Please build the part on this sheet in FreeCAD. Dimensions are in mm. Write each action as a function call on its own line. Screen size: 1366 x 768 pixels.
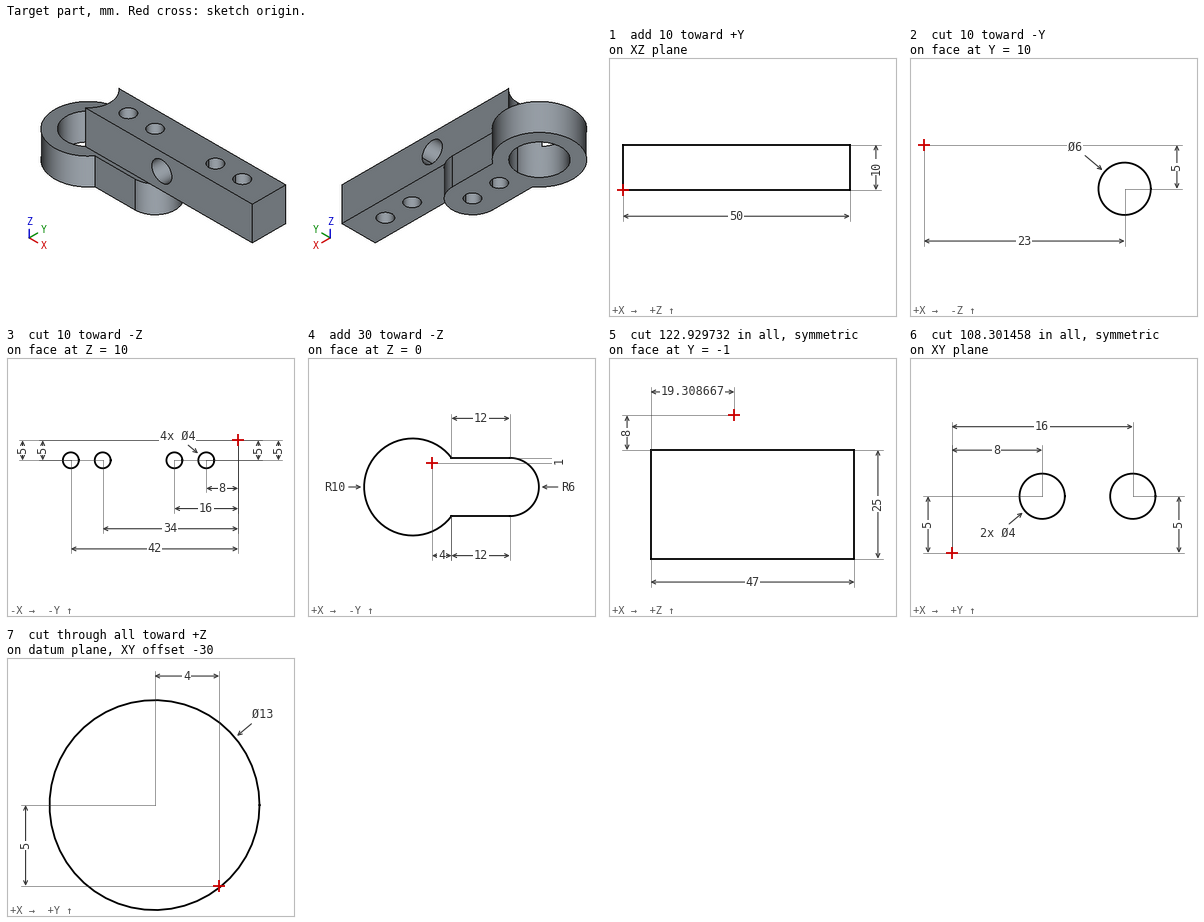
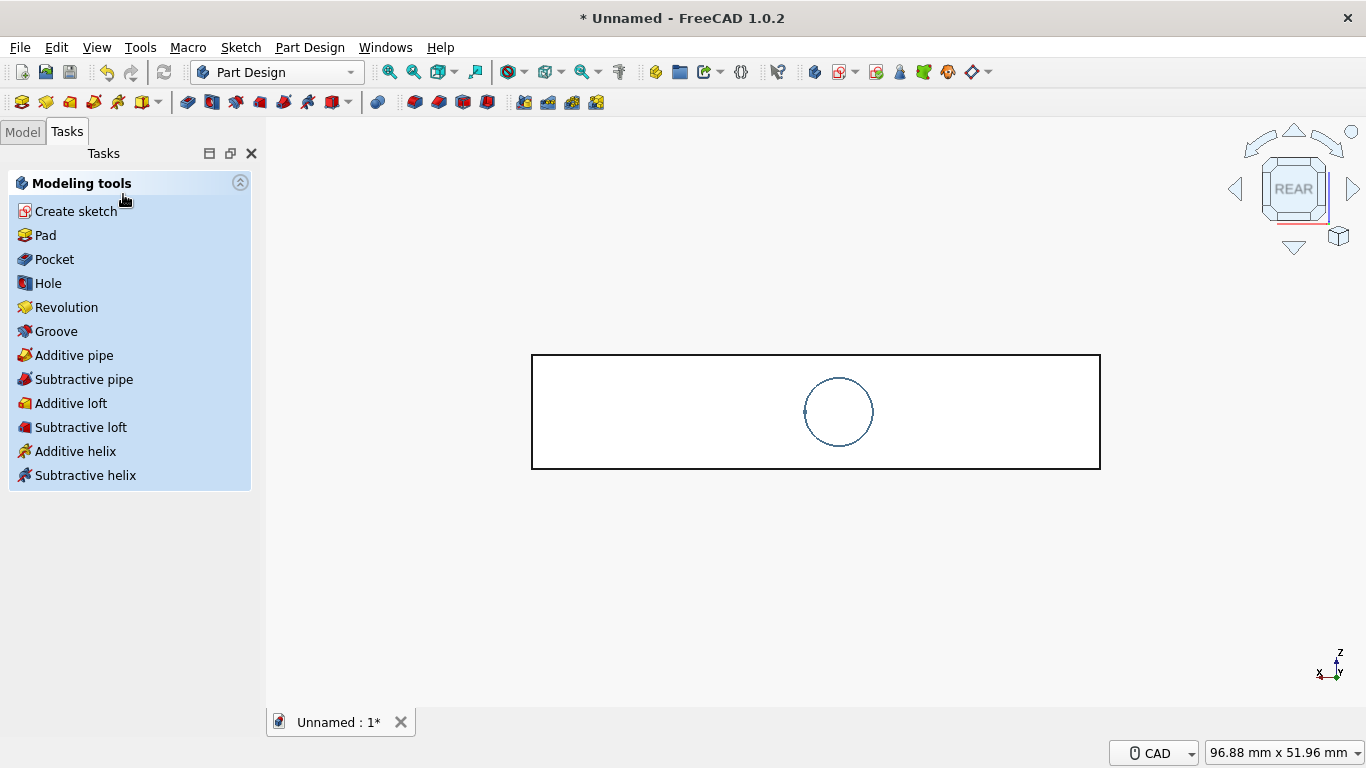
click(188, 102)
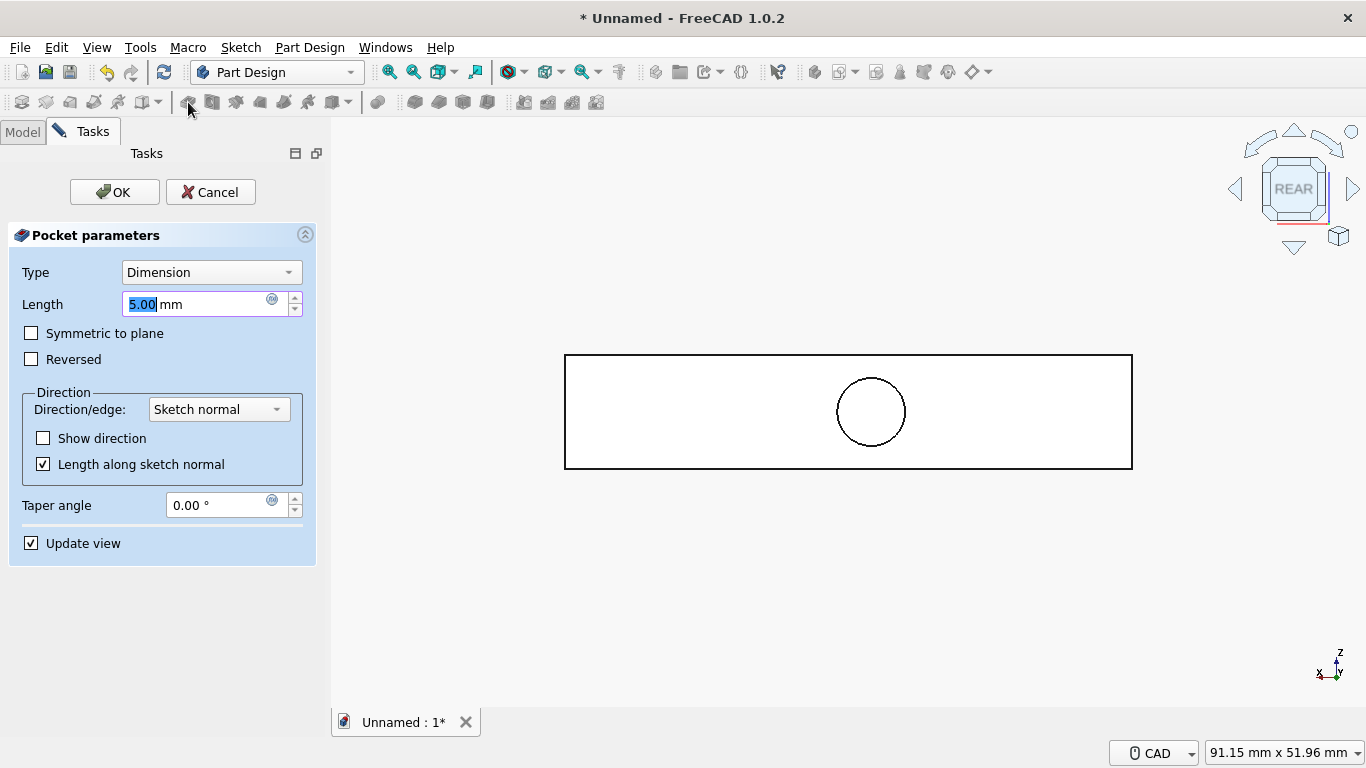
text(10)
key(Tab)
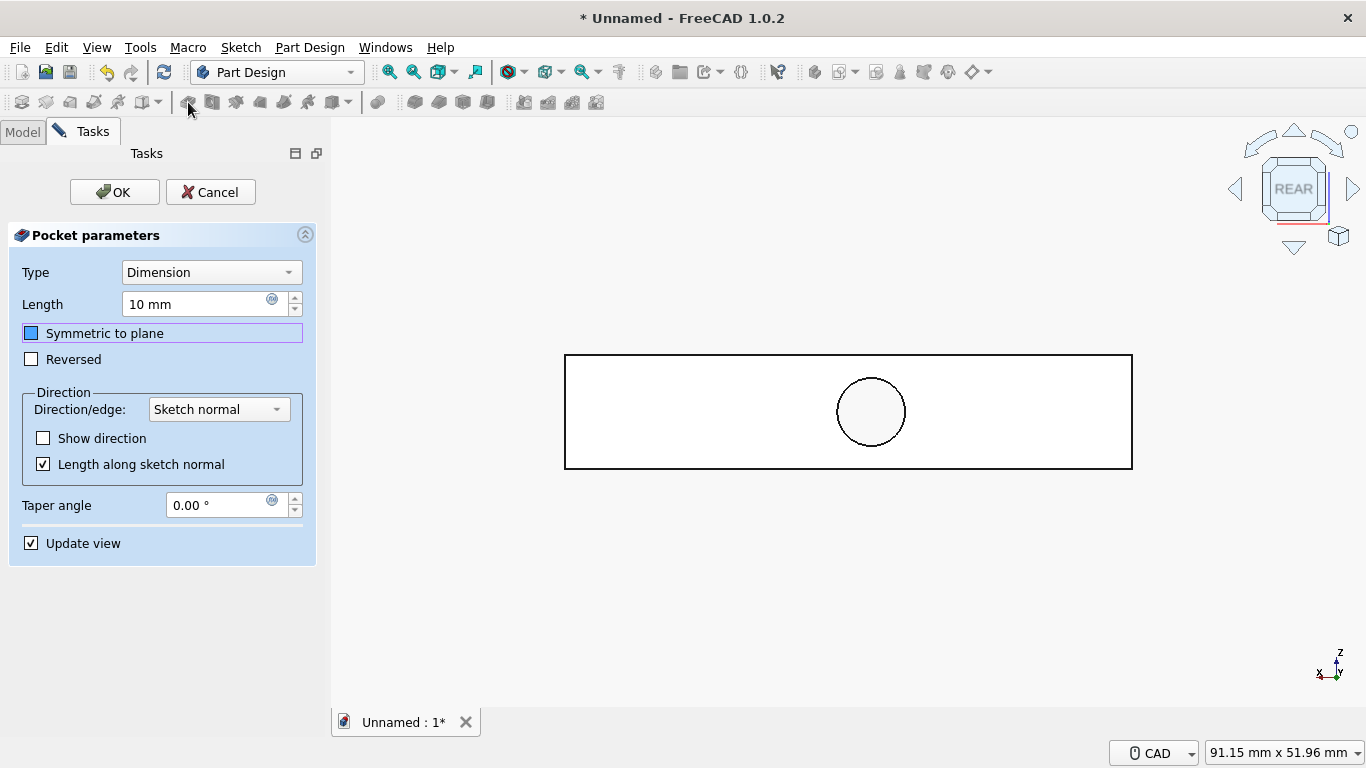
click(115, 192)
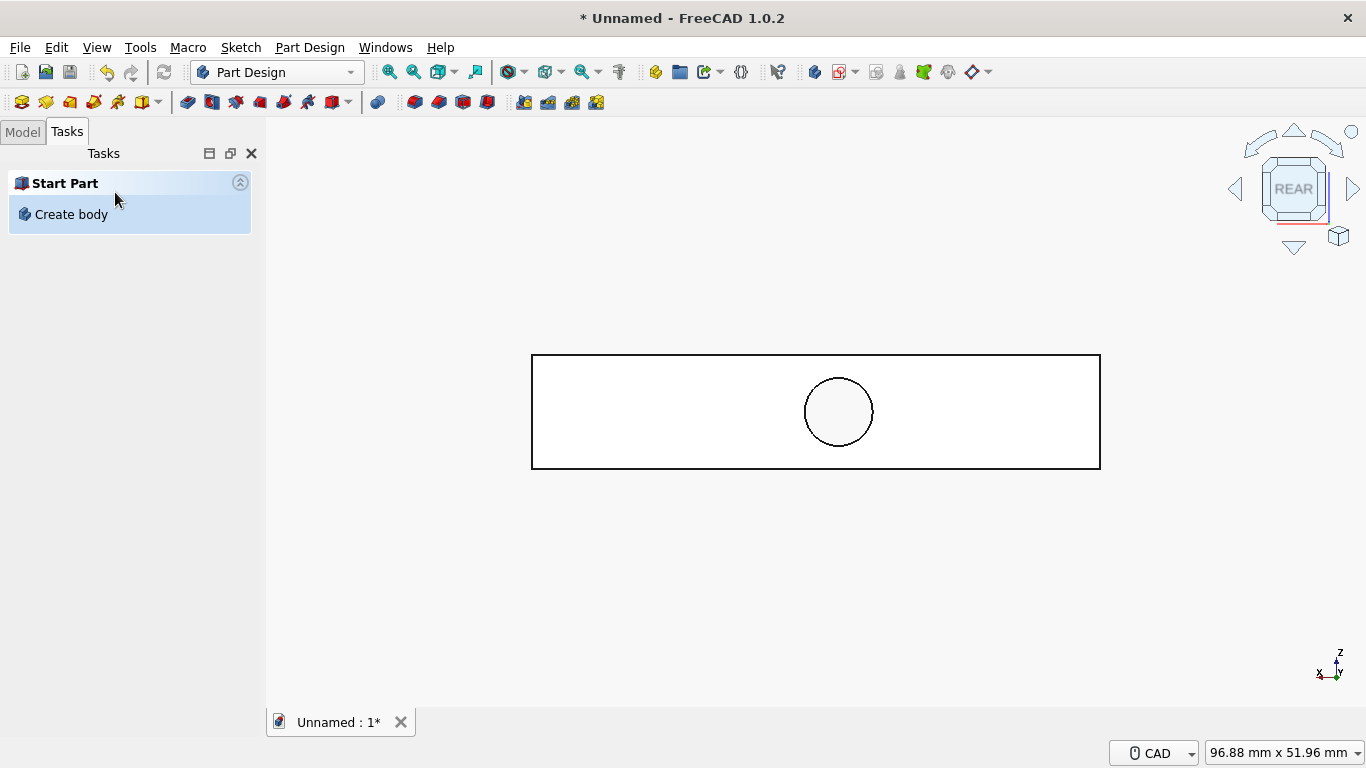
key(0)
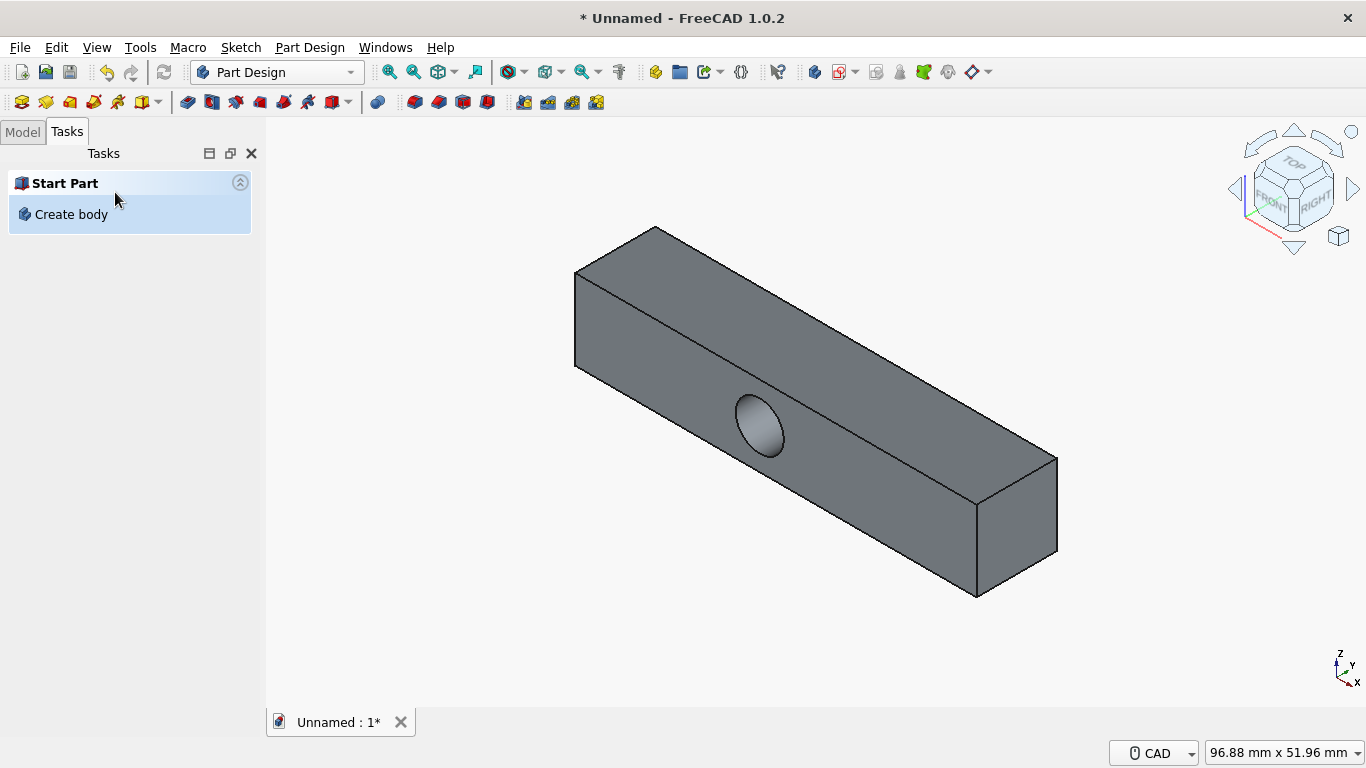
click(931, 431)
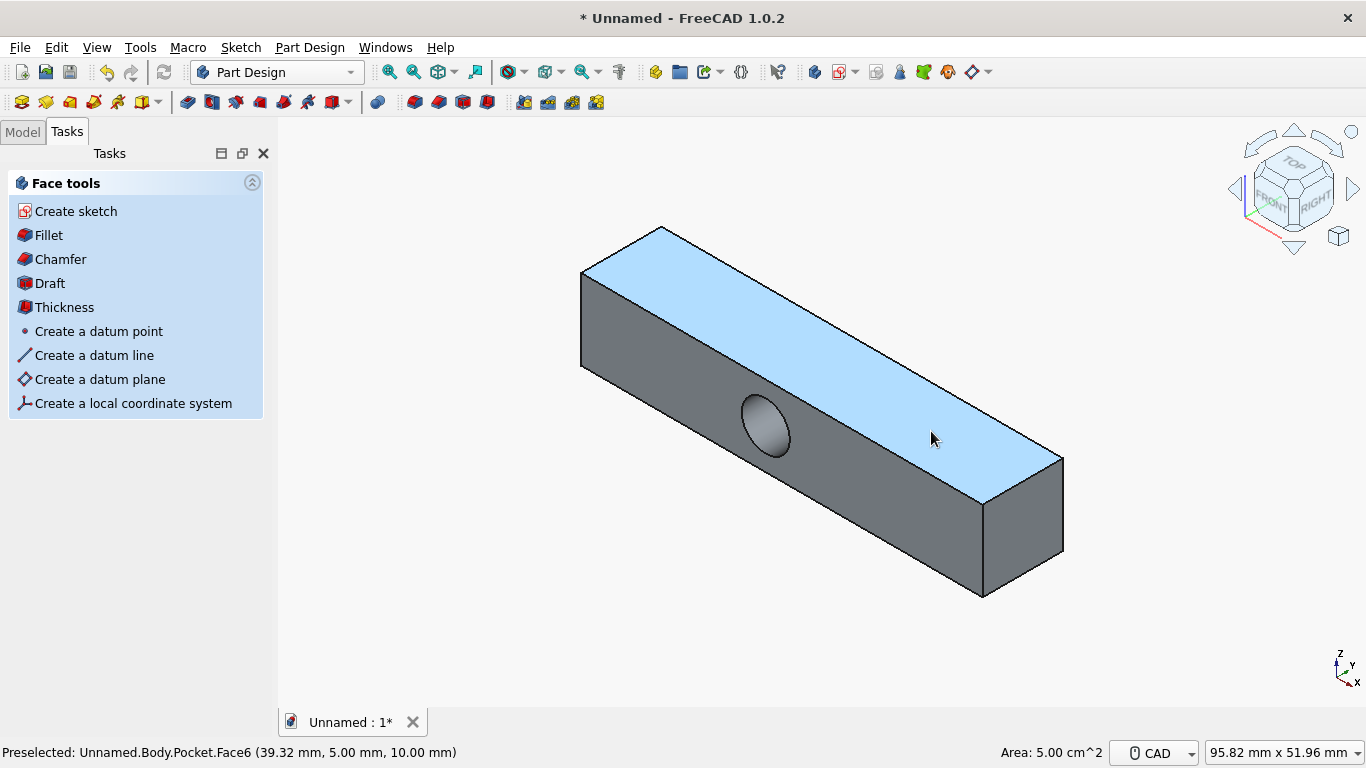
click(840, 72)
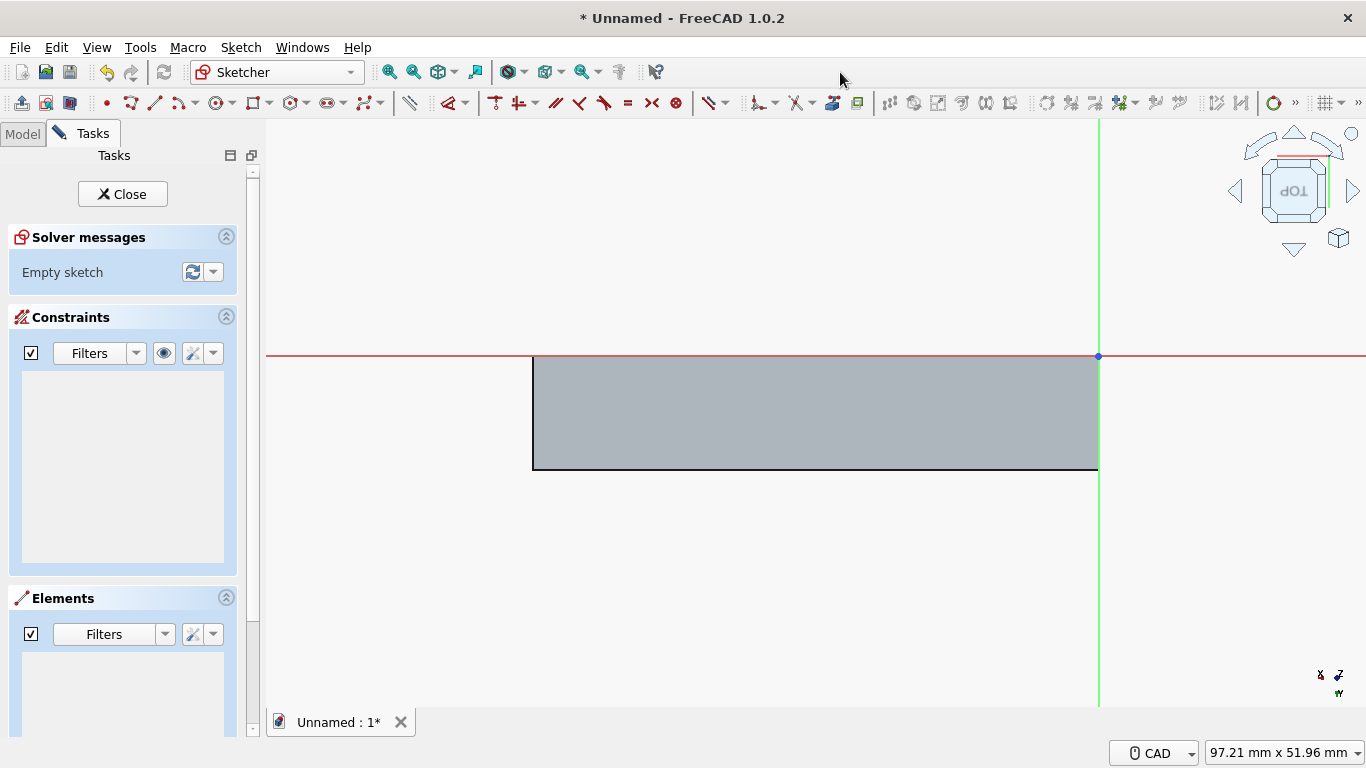
click(216, 104)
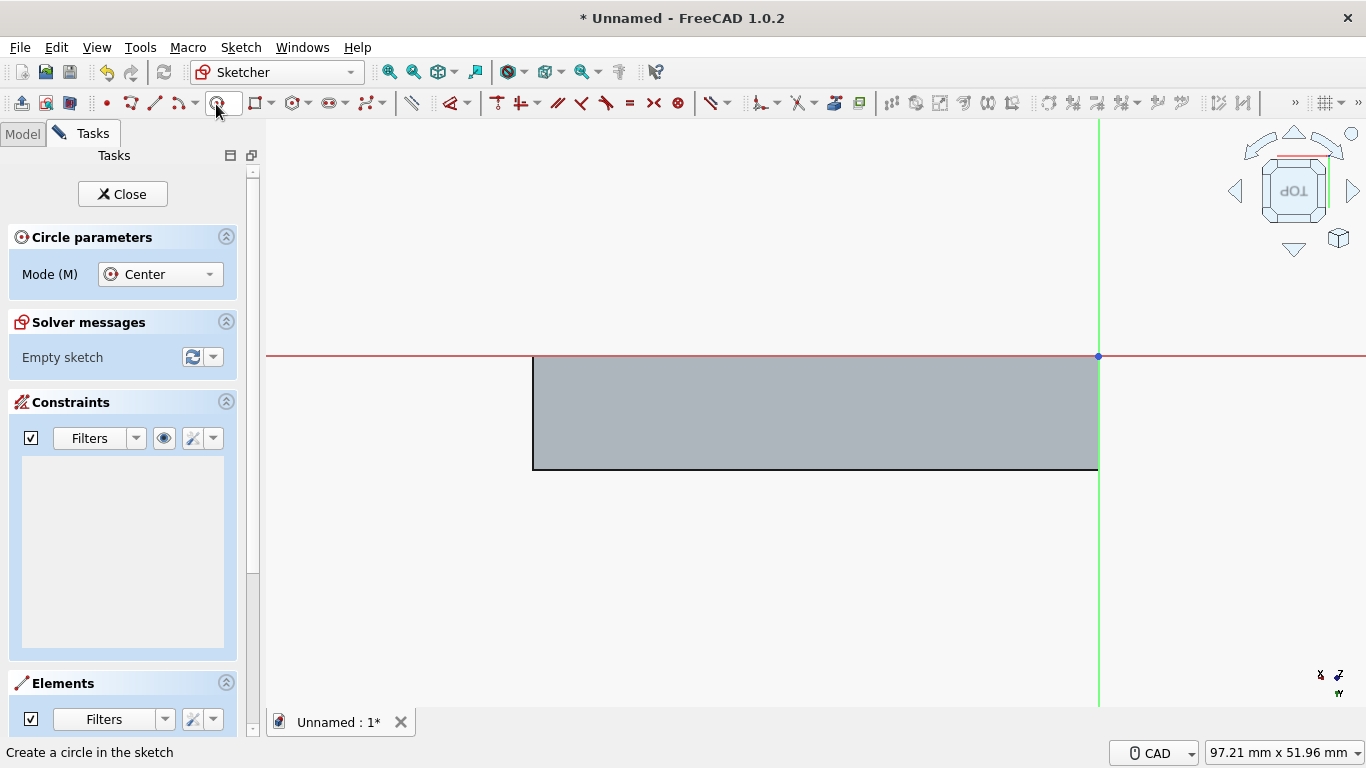
click(1008, 413)
move(1024, 397)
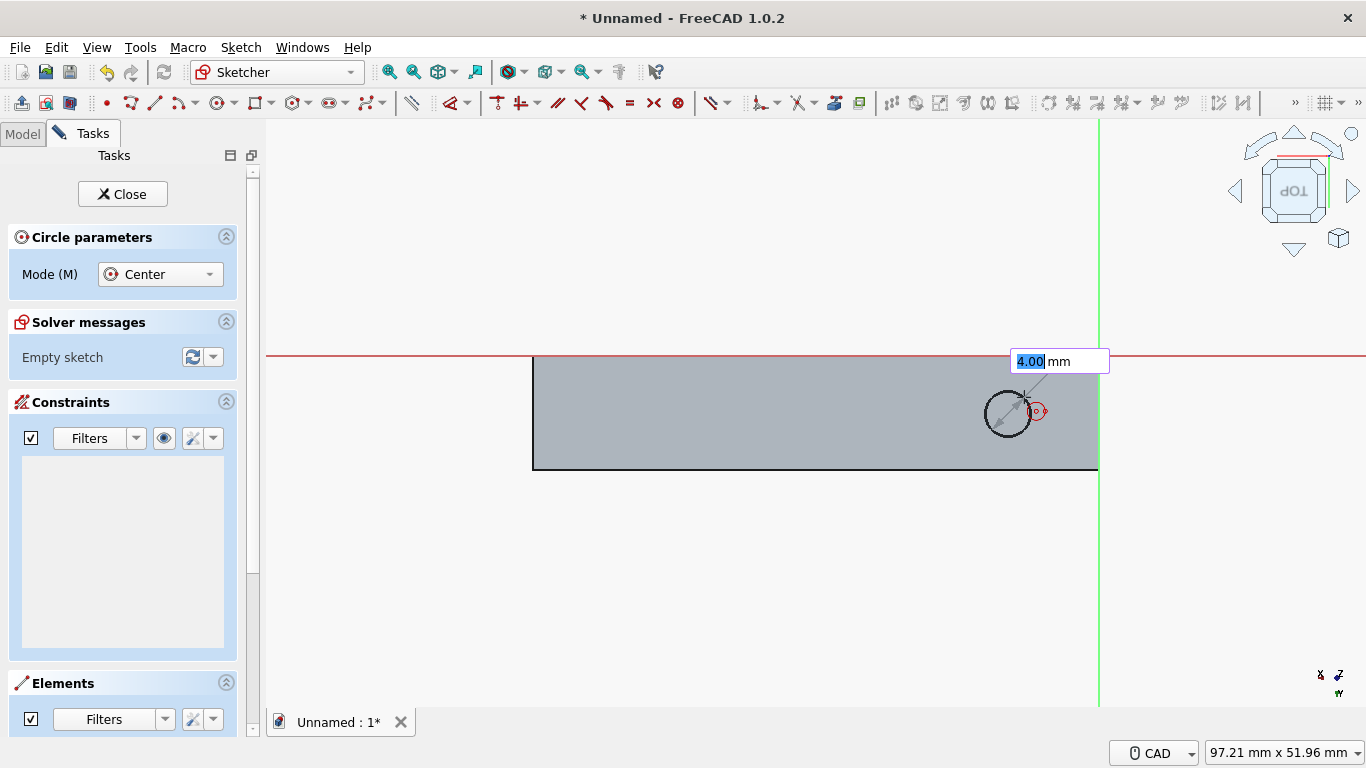
text(4)
key(Return)